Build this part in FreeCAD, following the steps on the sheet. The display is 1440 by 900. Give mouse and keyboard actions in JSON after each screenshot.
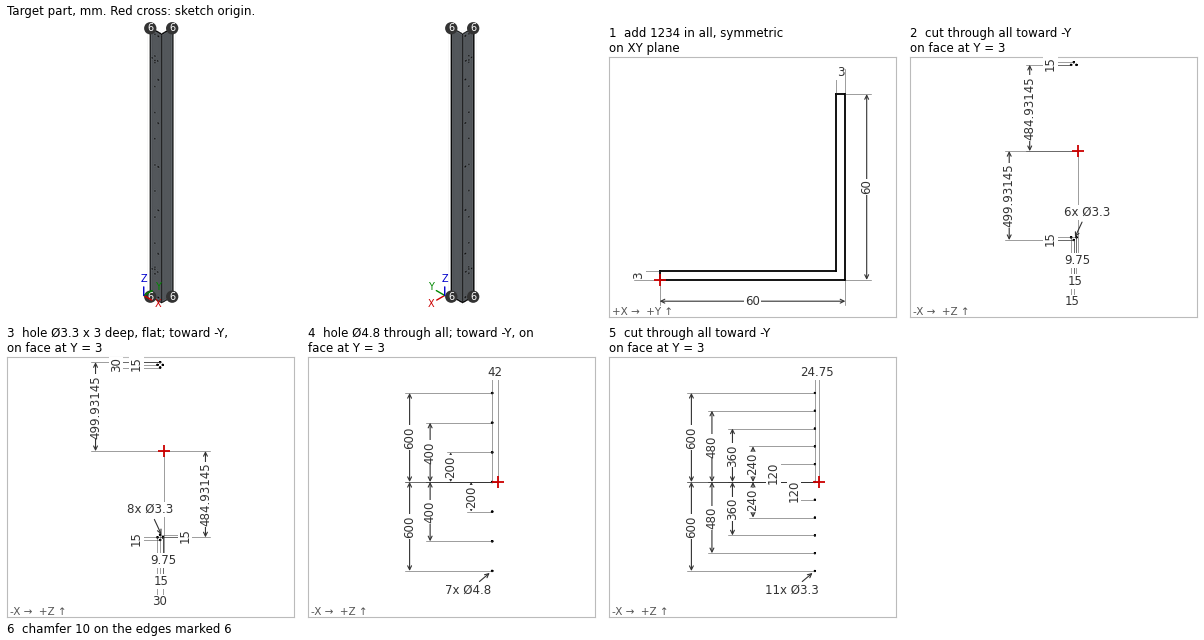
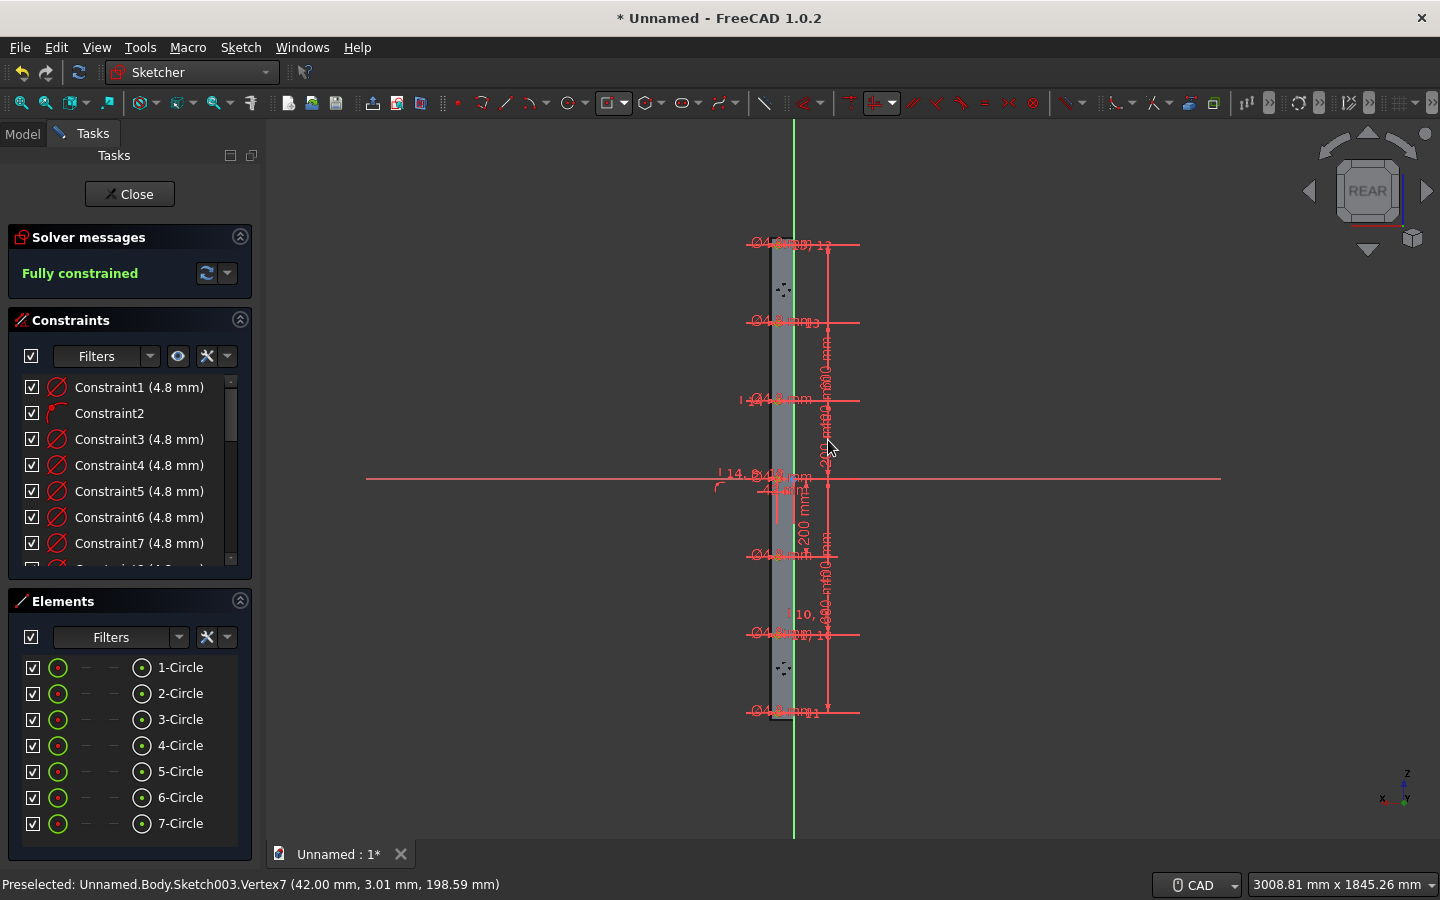
{"action": "left_click", "coordinate": [130, 194]}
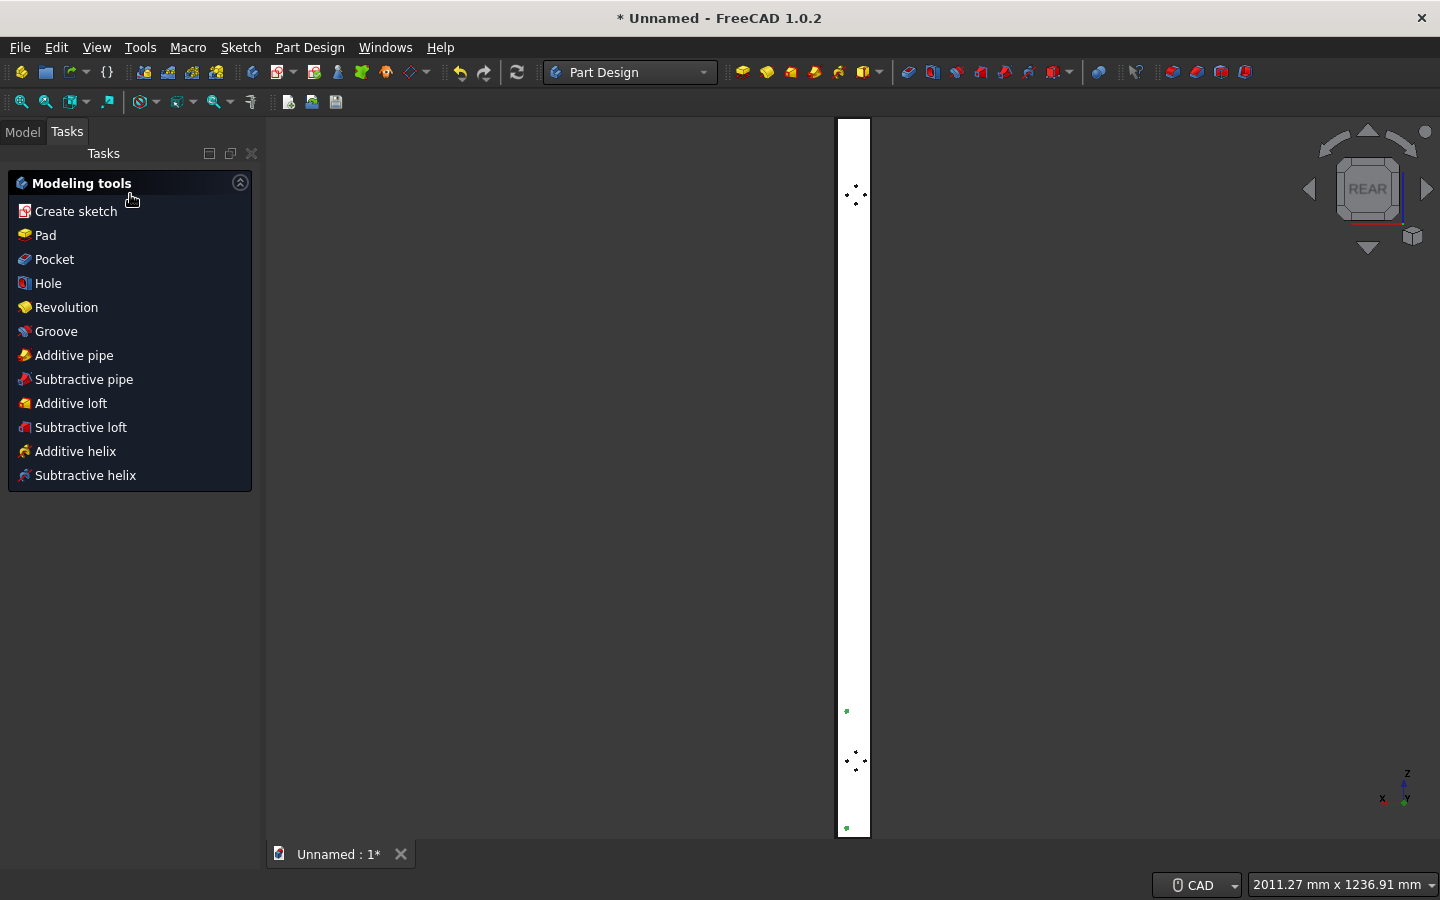
{"action": "left_click", "coordinate": [934, 72]}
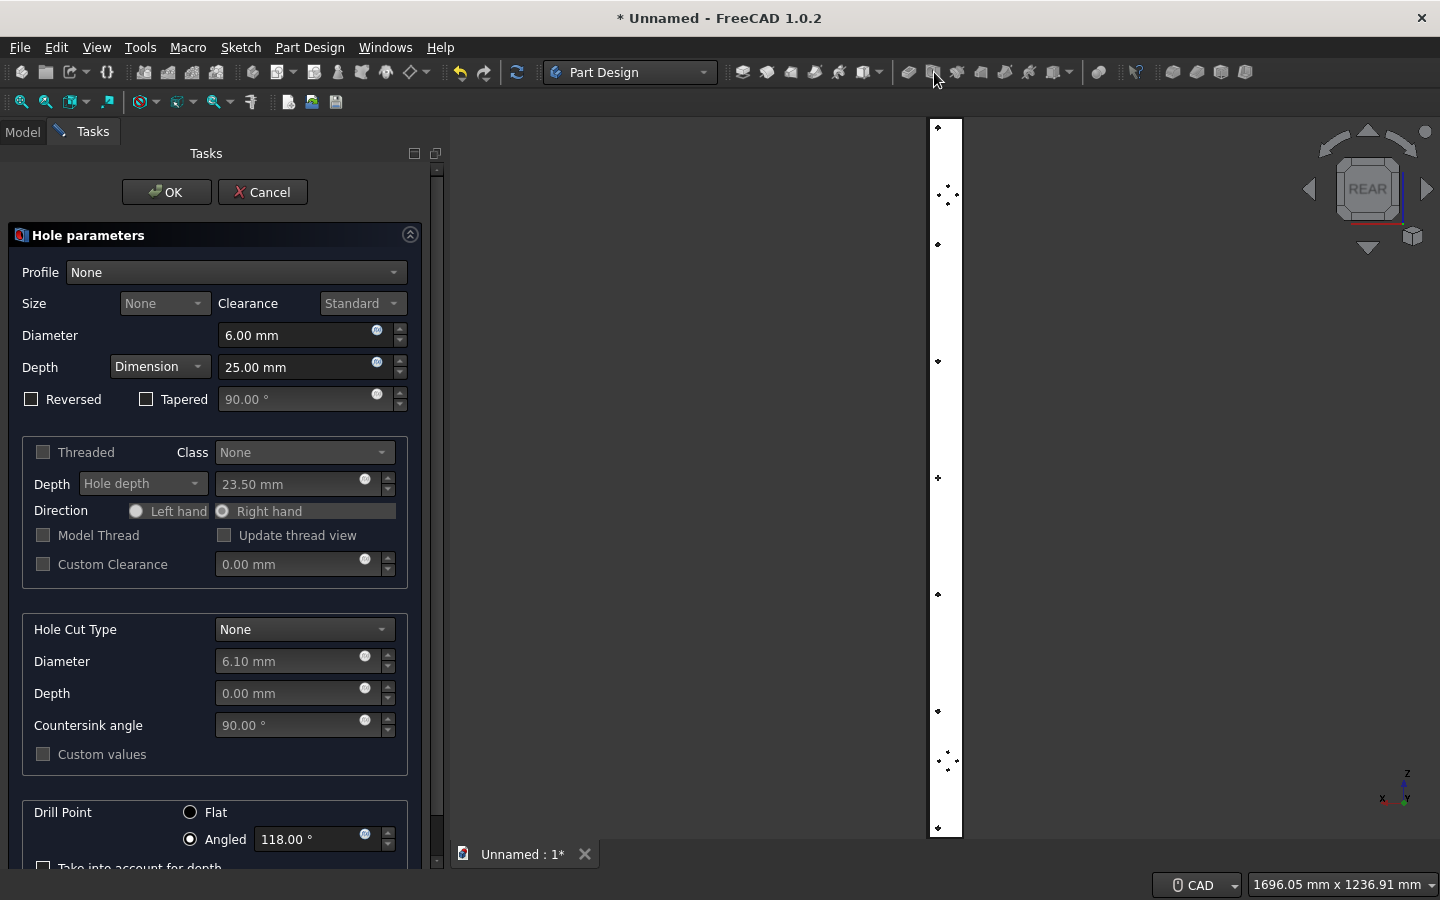
{"action": "triple_click", "coordinate": [305, 335]}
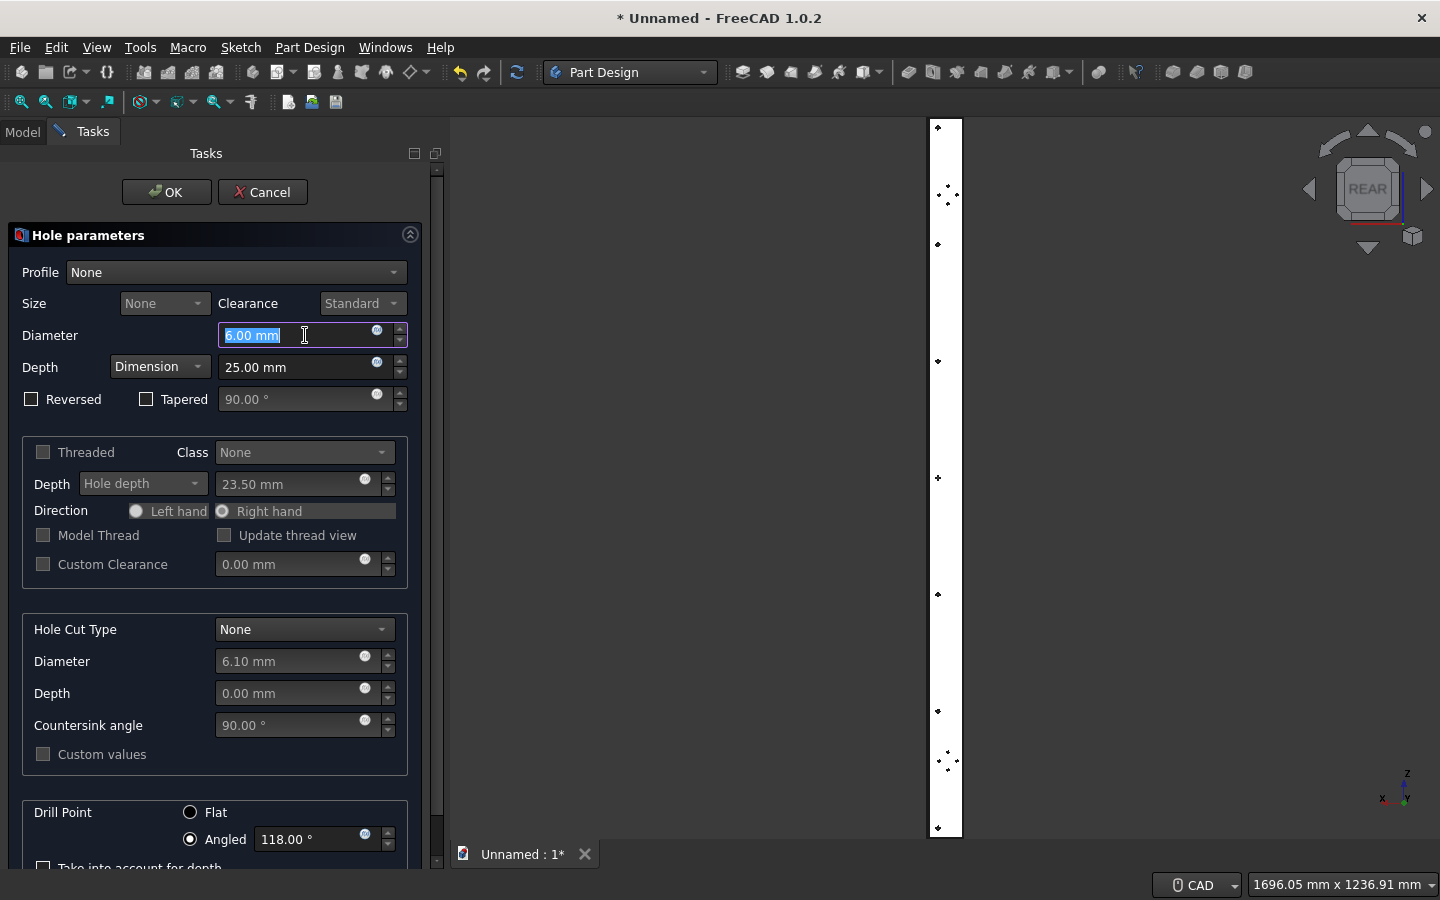
{"action": "type", "text": "4.8"}
{"action": "key", "text": "Tab"}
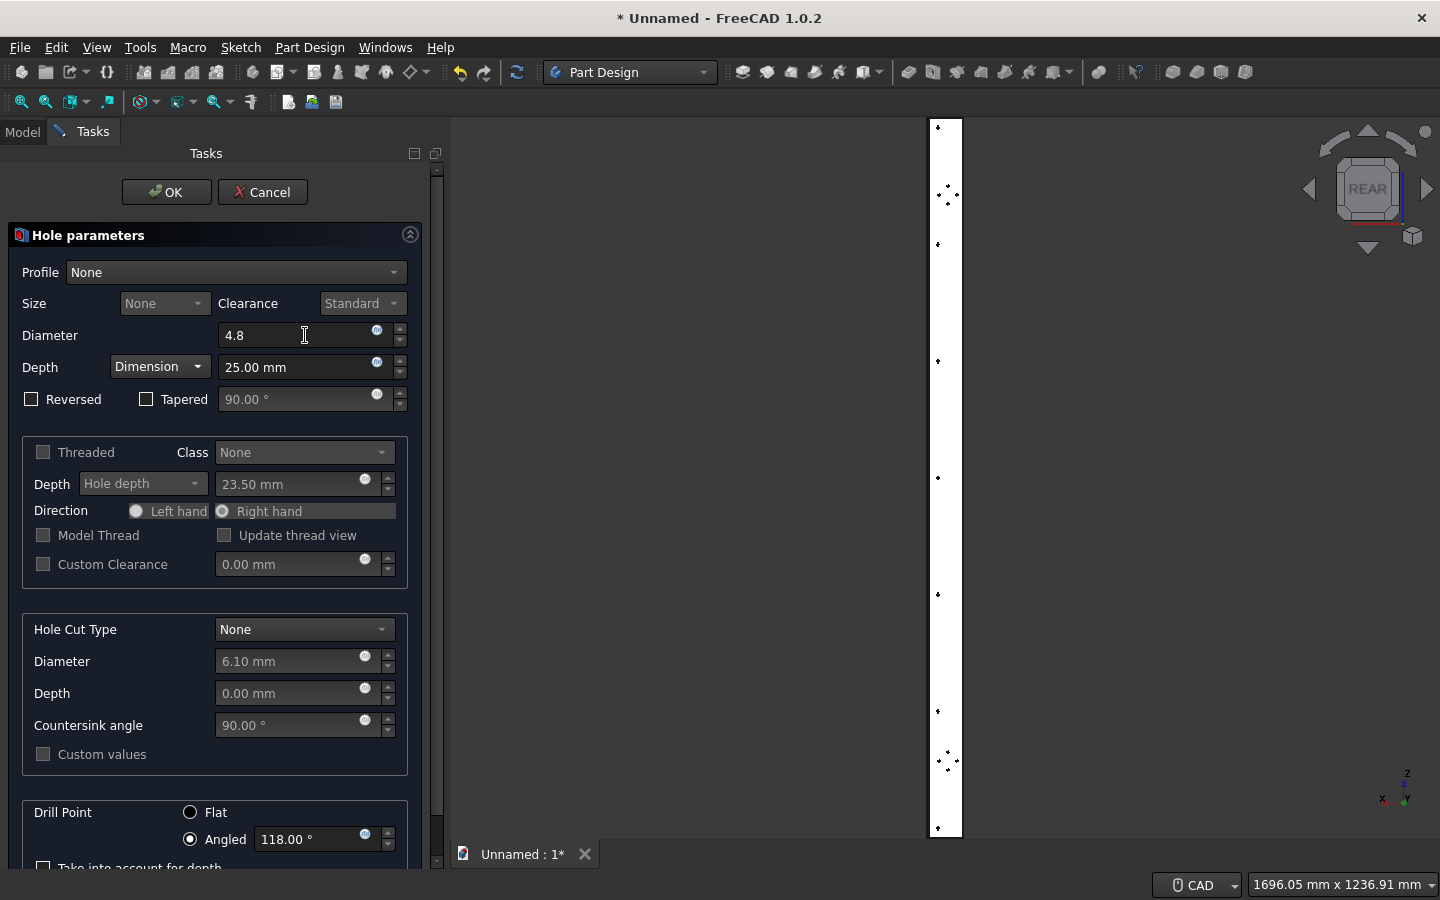
{"action": "left_click", "coordinate": [161, 366]}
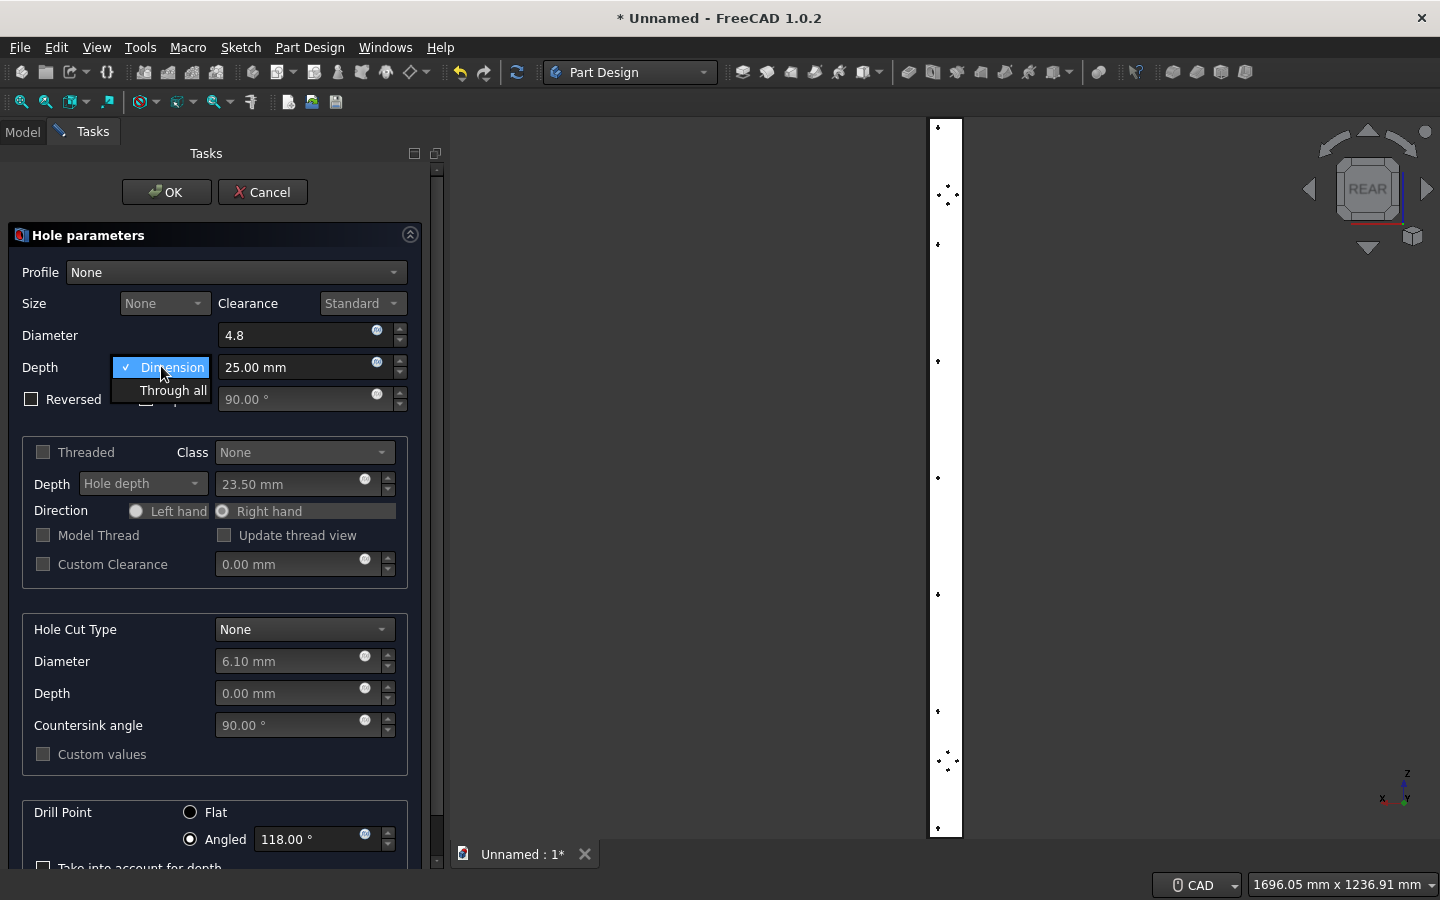
{"action": "left_click", "coordinate": [160, 390]}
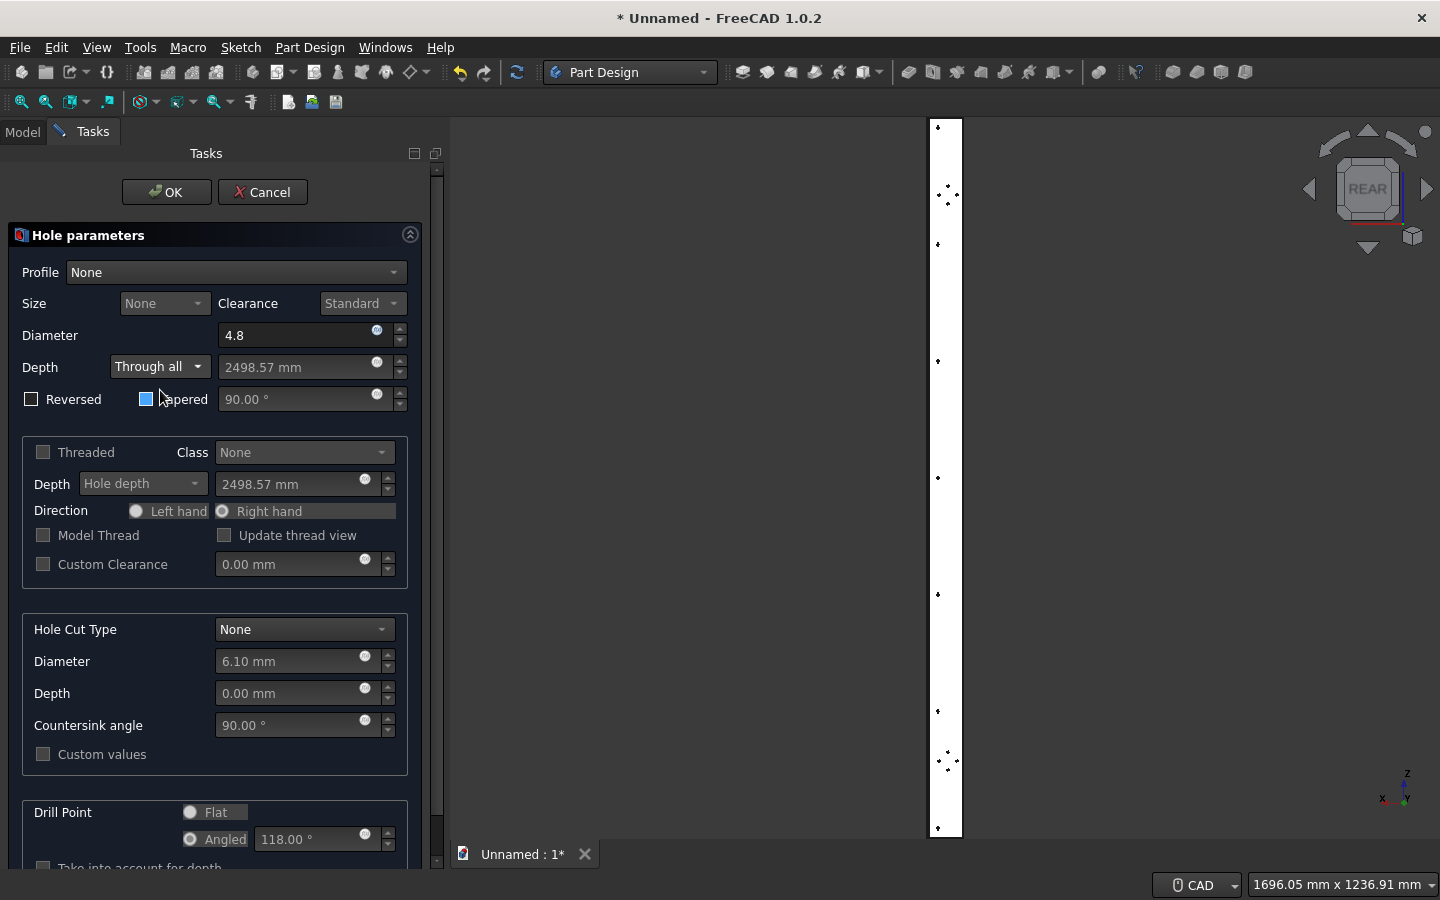
{"action": "left_click", "coordinate": [167, 192]}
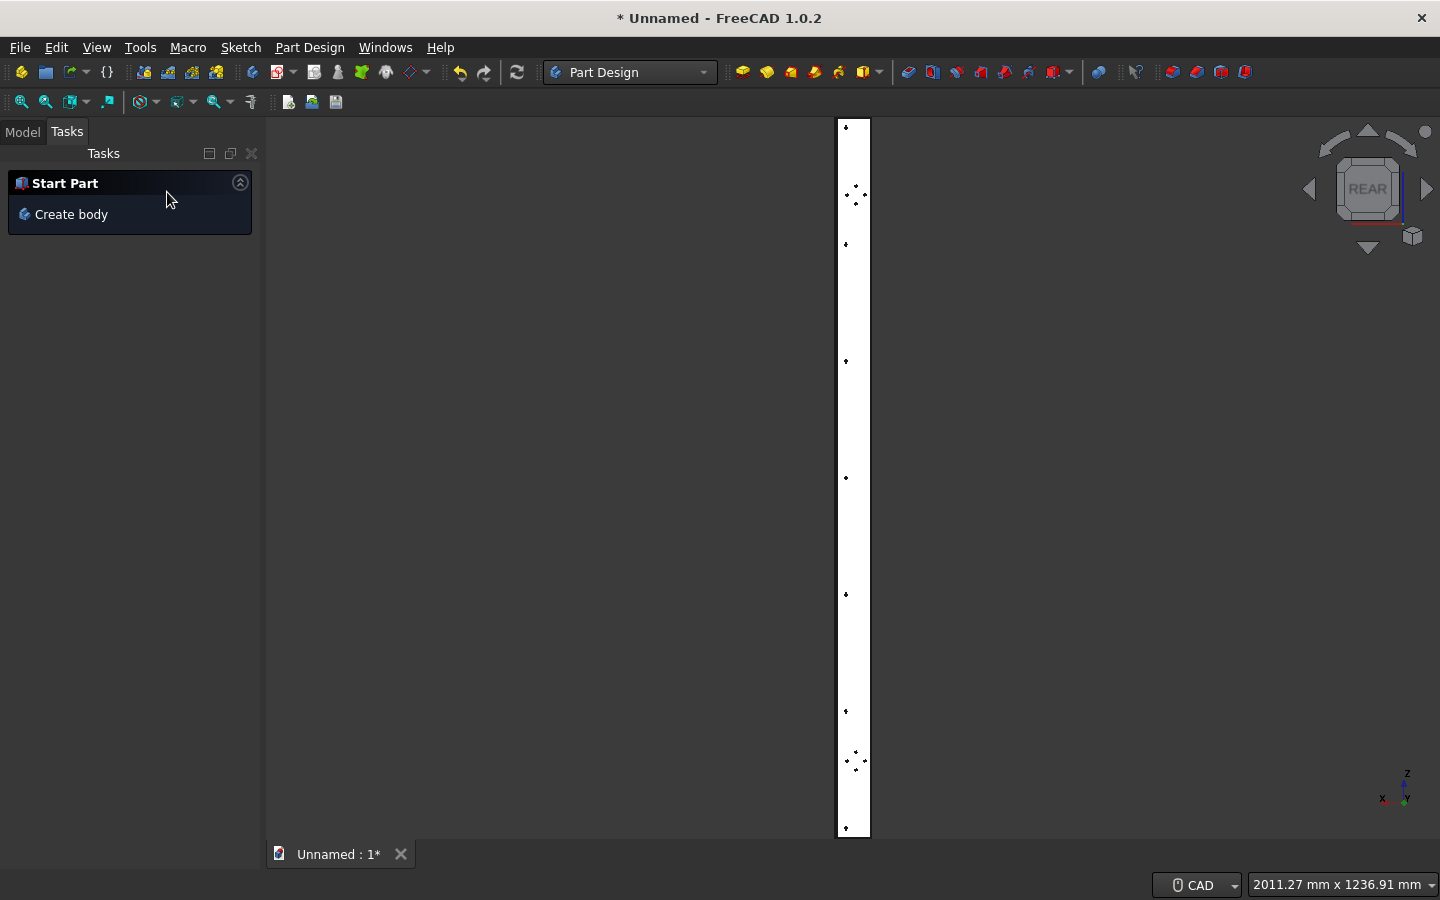
{"action": "left_click", "coordinate": [854, 271]}